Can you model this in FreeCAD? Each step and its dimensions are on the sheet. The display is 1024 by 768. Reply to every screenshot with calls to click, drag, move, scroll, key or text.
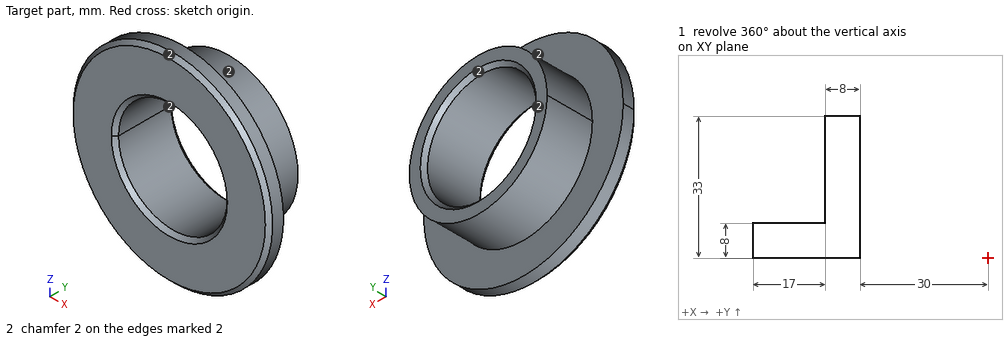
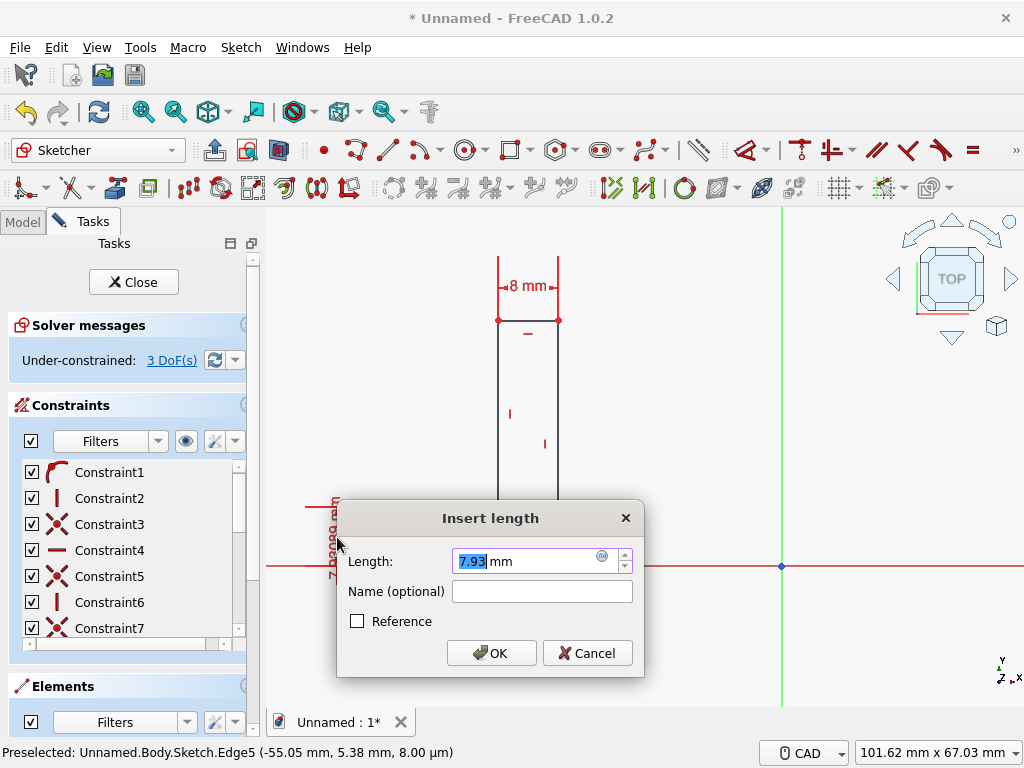
text(8)
key(Return)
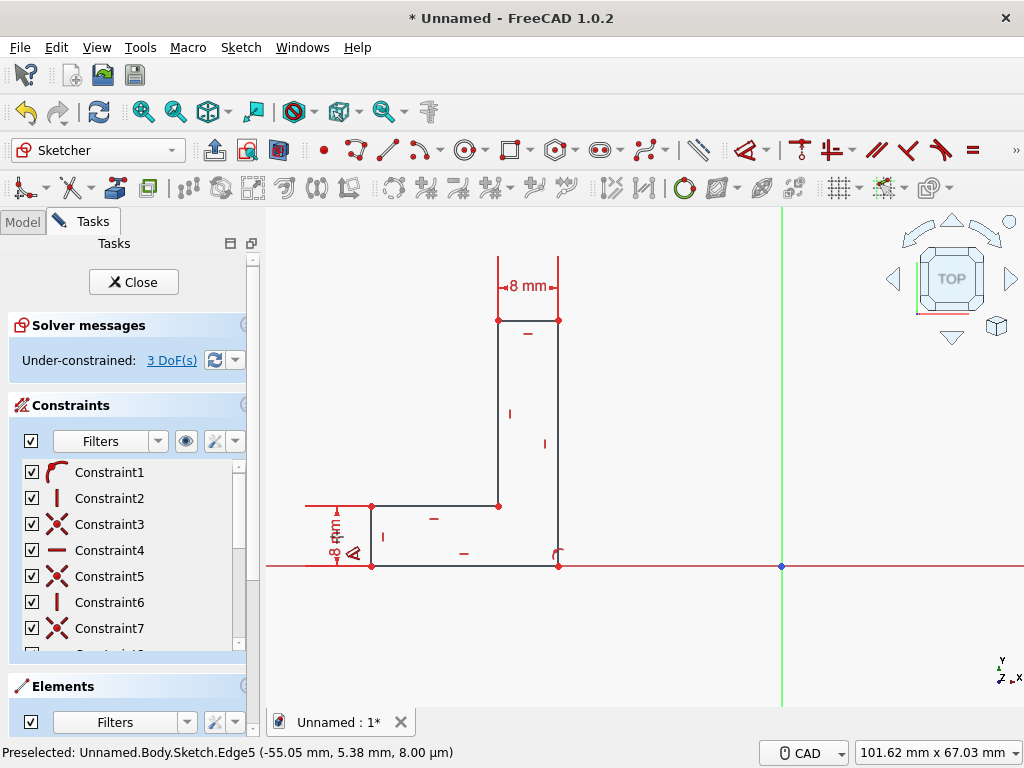
click(558, 493)
click(524, 444)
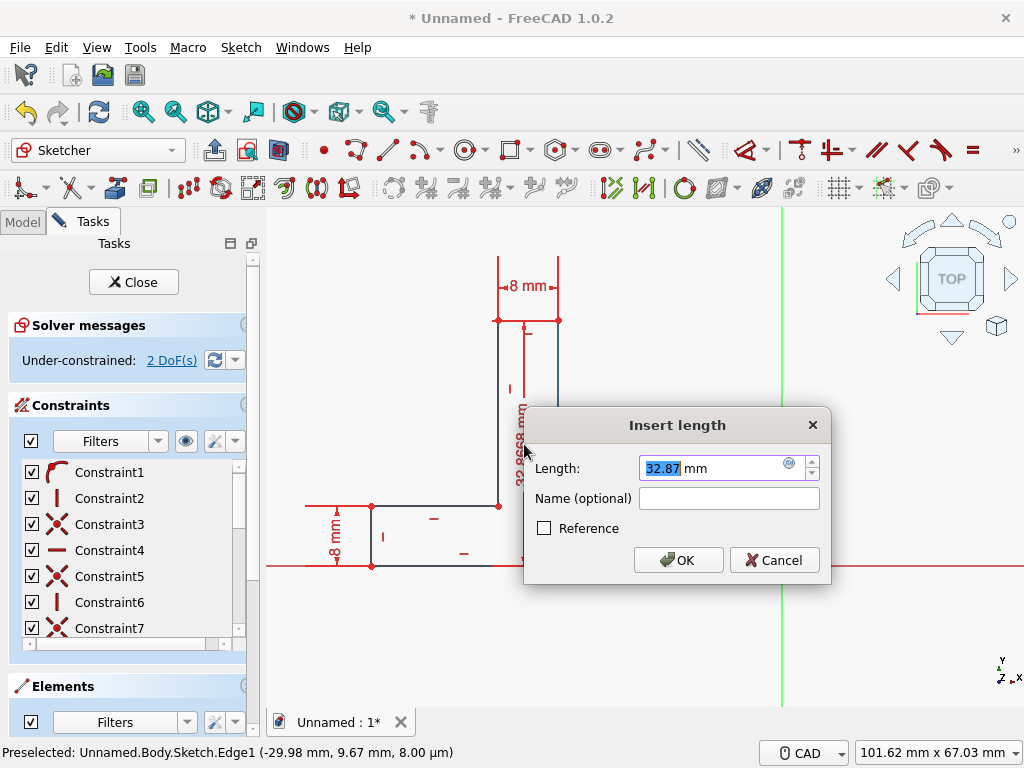
text(33)
key(Return)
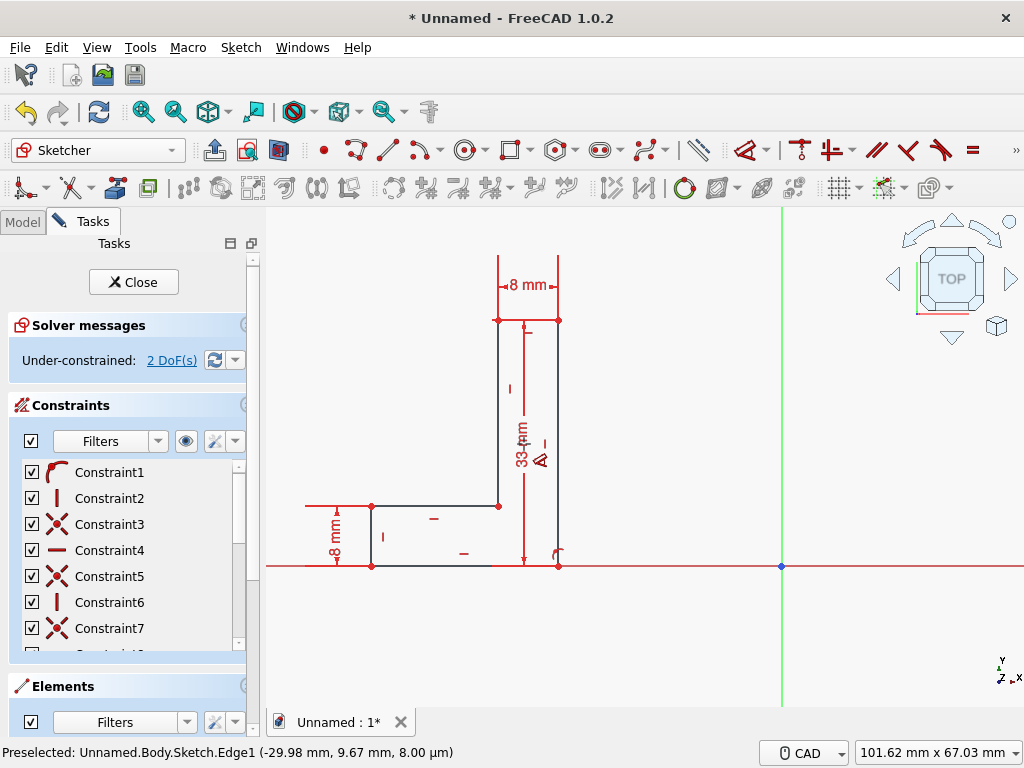
click(460, 506)
click(435, 540)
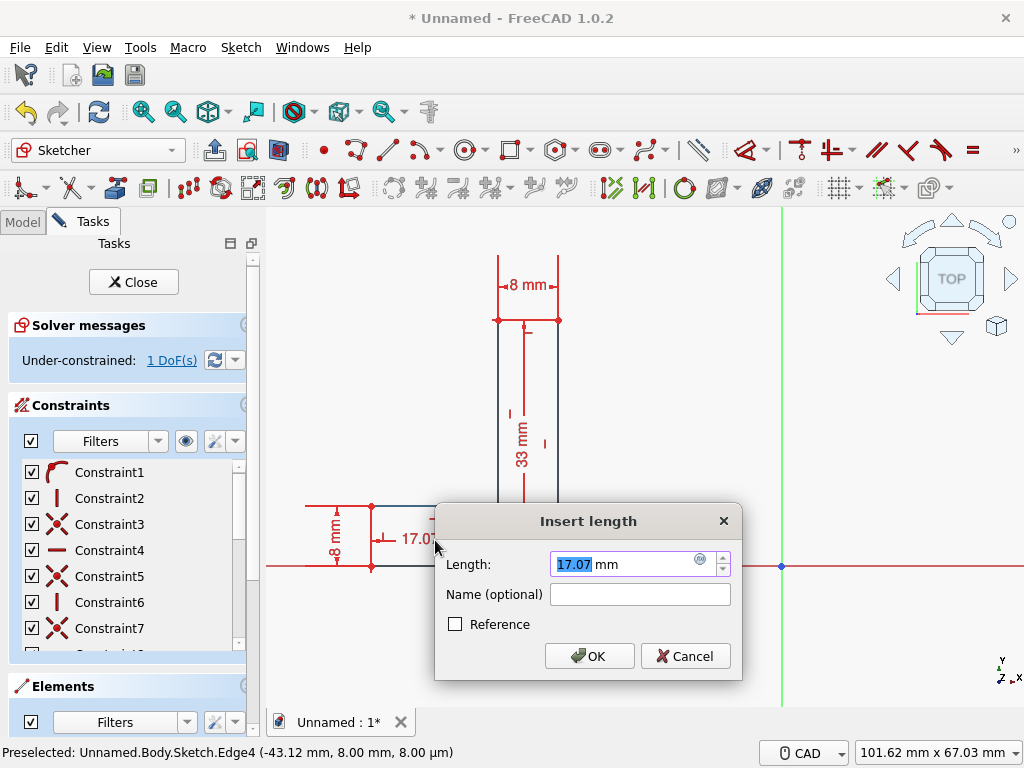
text(17)
key(Return)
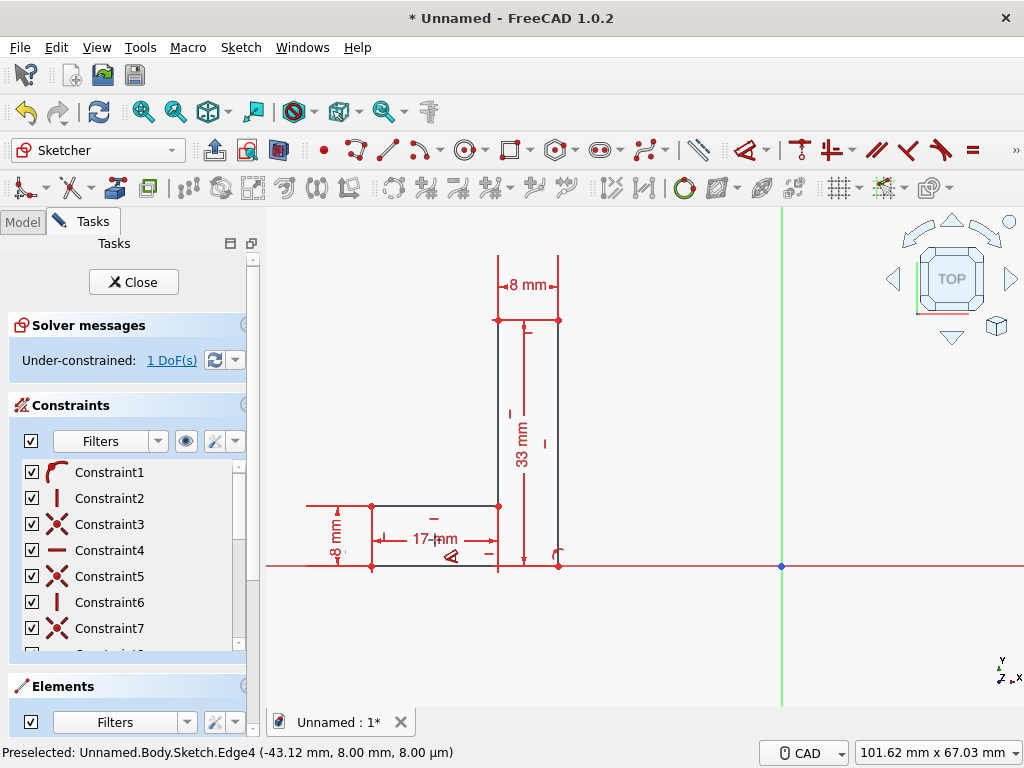
click(558, 566)
click(670, 600)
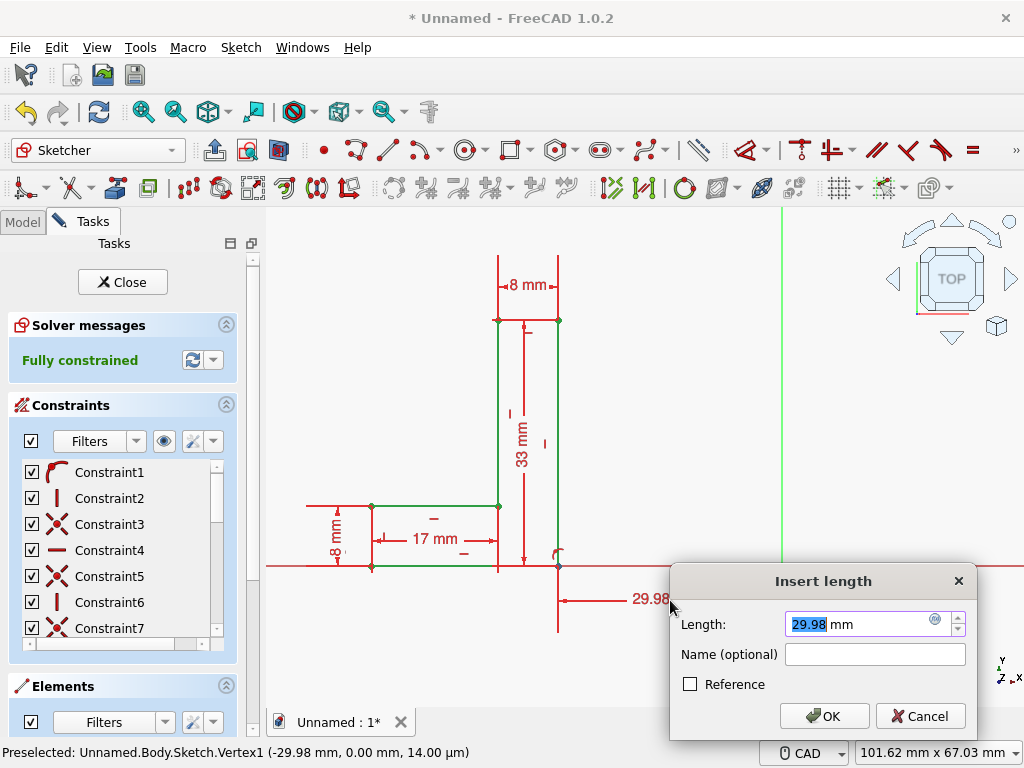
text(30)
key(Return)
key(Escape)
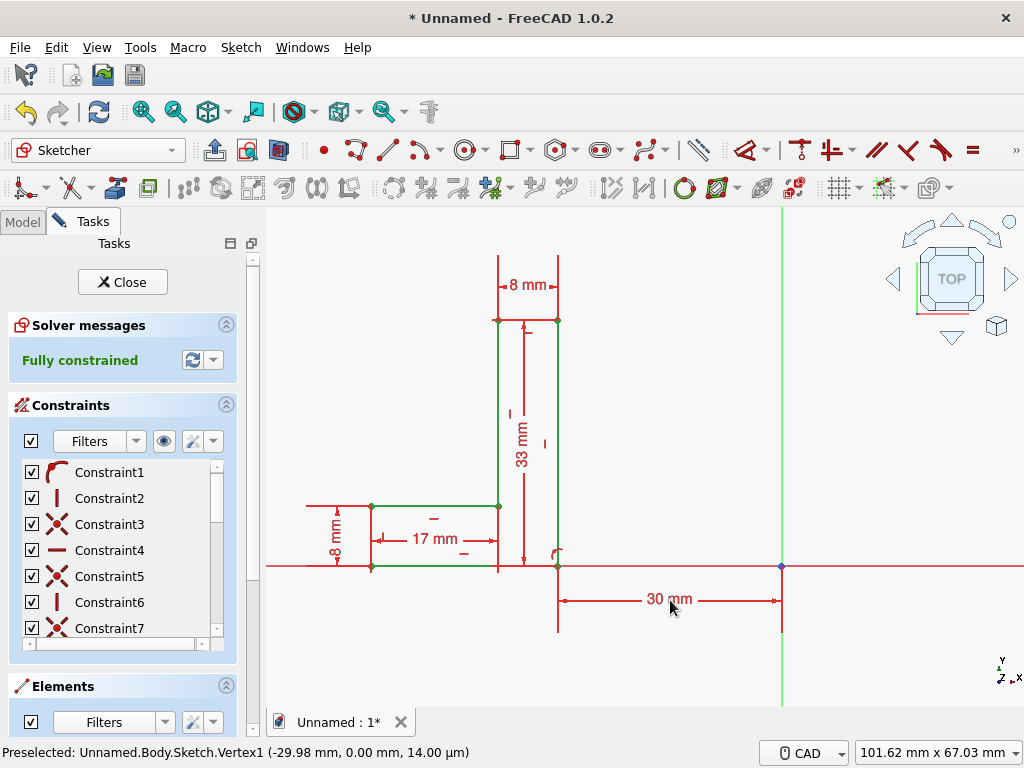
click(123, 282)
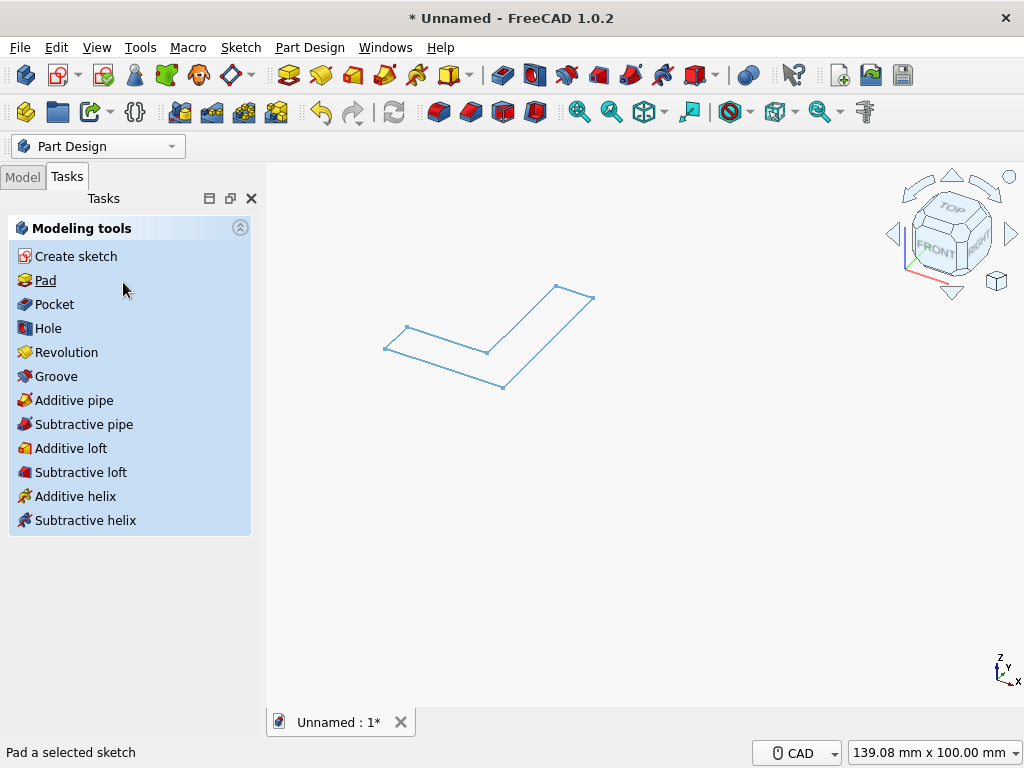
click(322, 76)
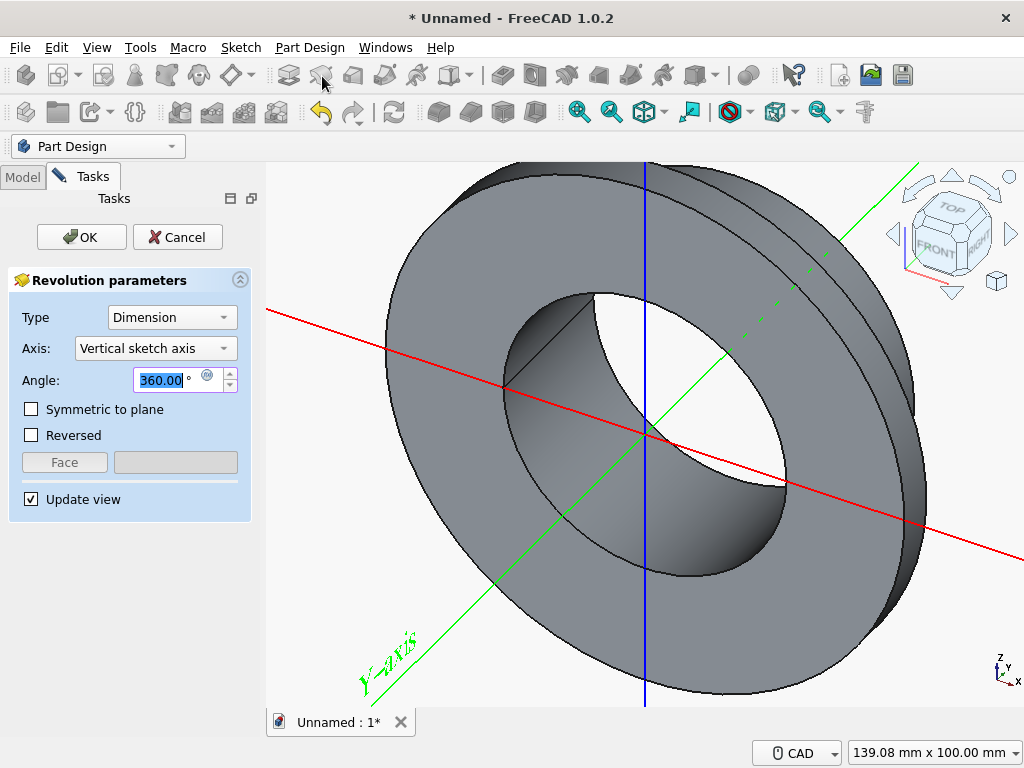
click(82, 237)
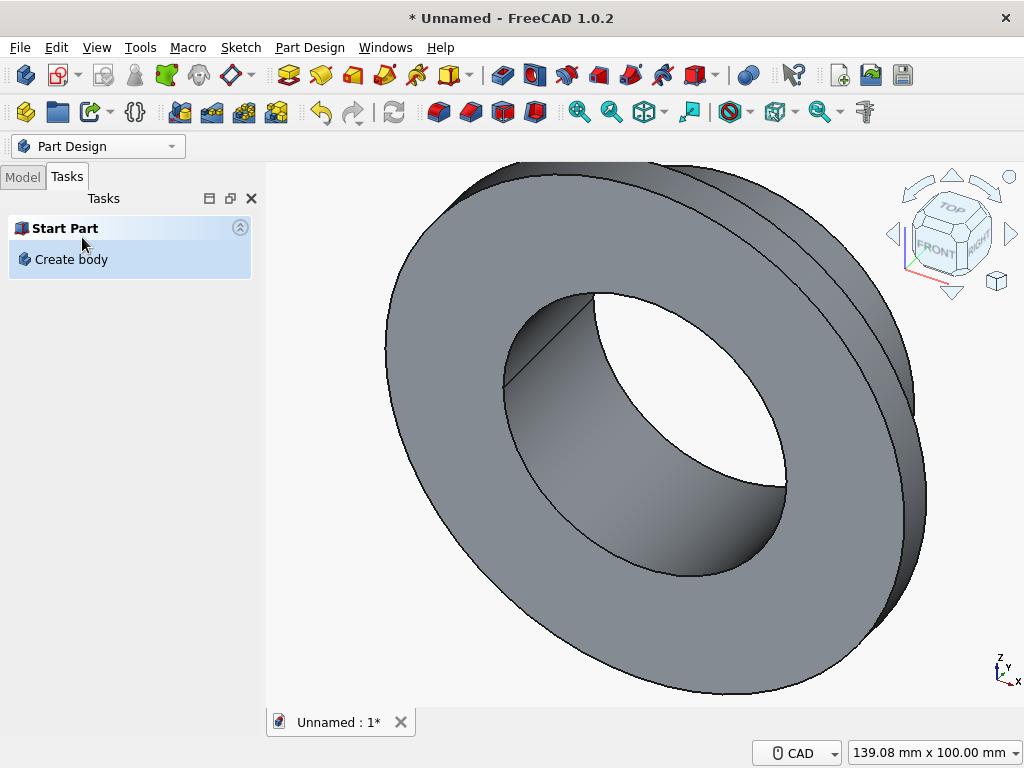
click(580, 112)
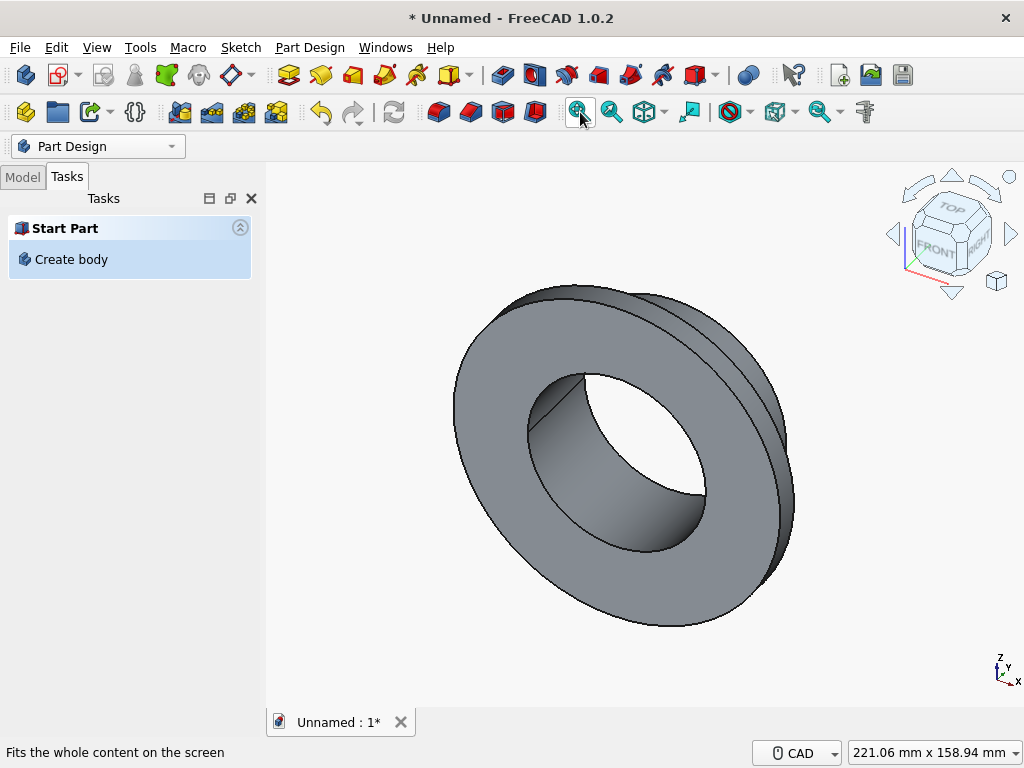
click(780, 516)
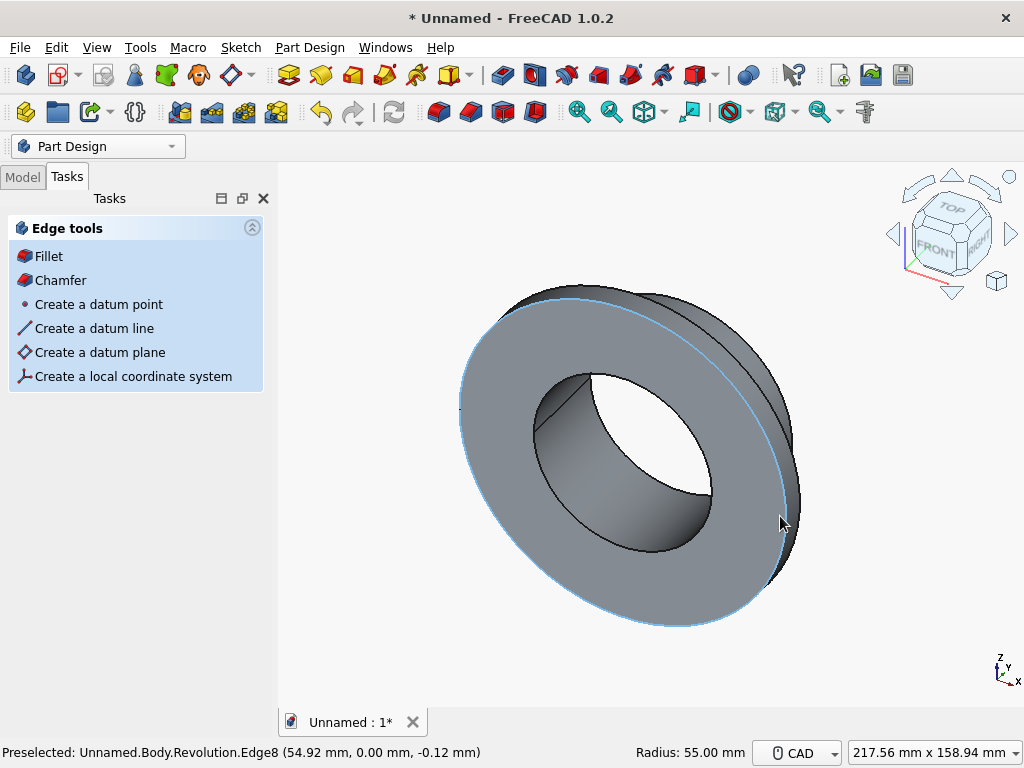
click(695, 535, ctrl)